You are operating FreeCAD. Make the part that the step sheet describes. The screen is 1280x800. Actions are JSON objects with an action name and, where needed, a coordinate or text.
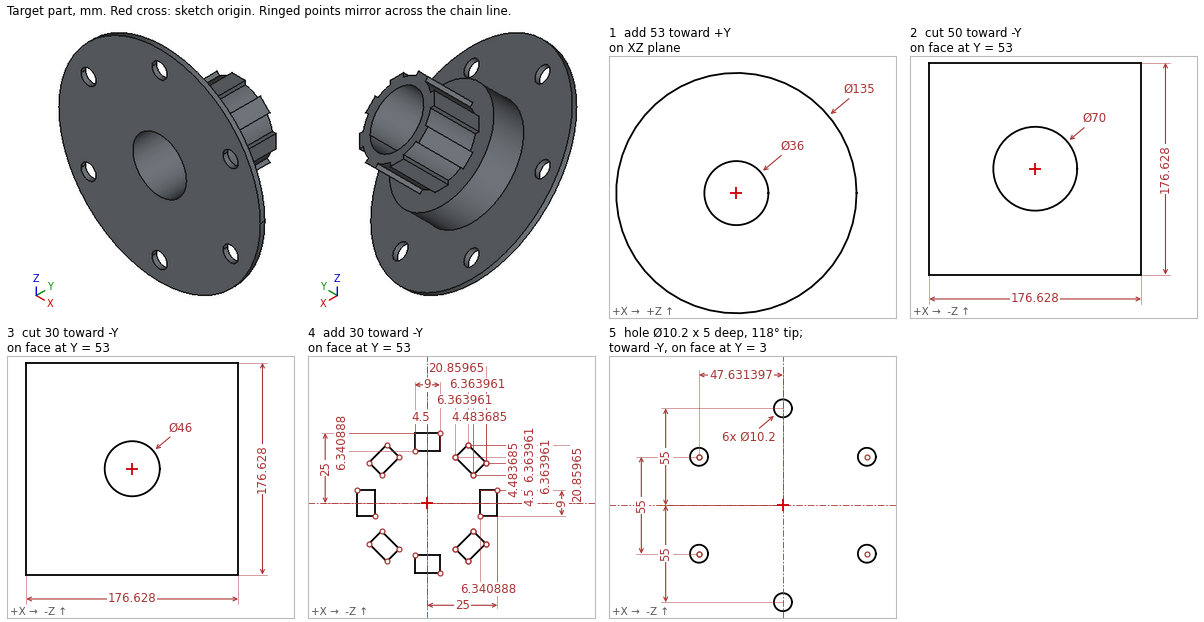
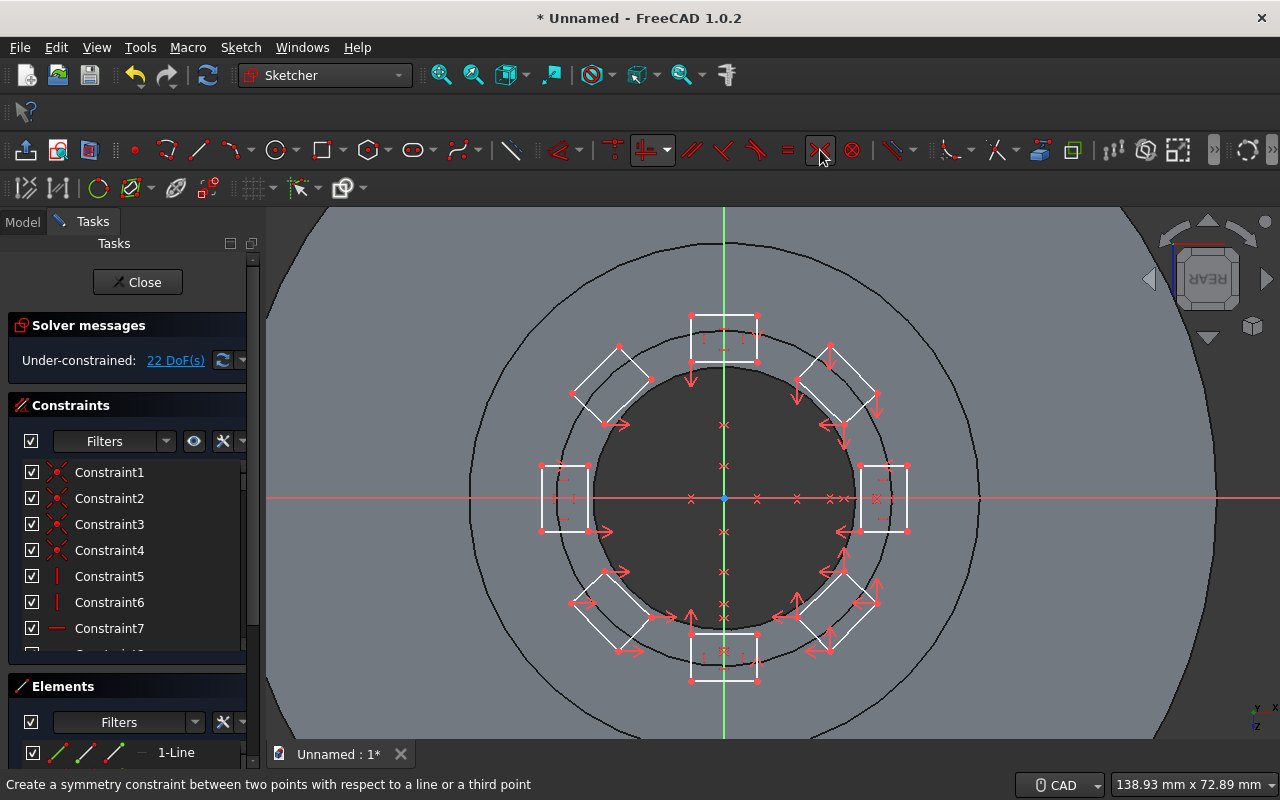
{"action": "left_click", "coordinate": [797, 379]}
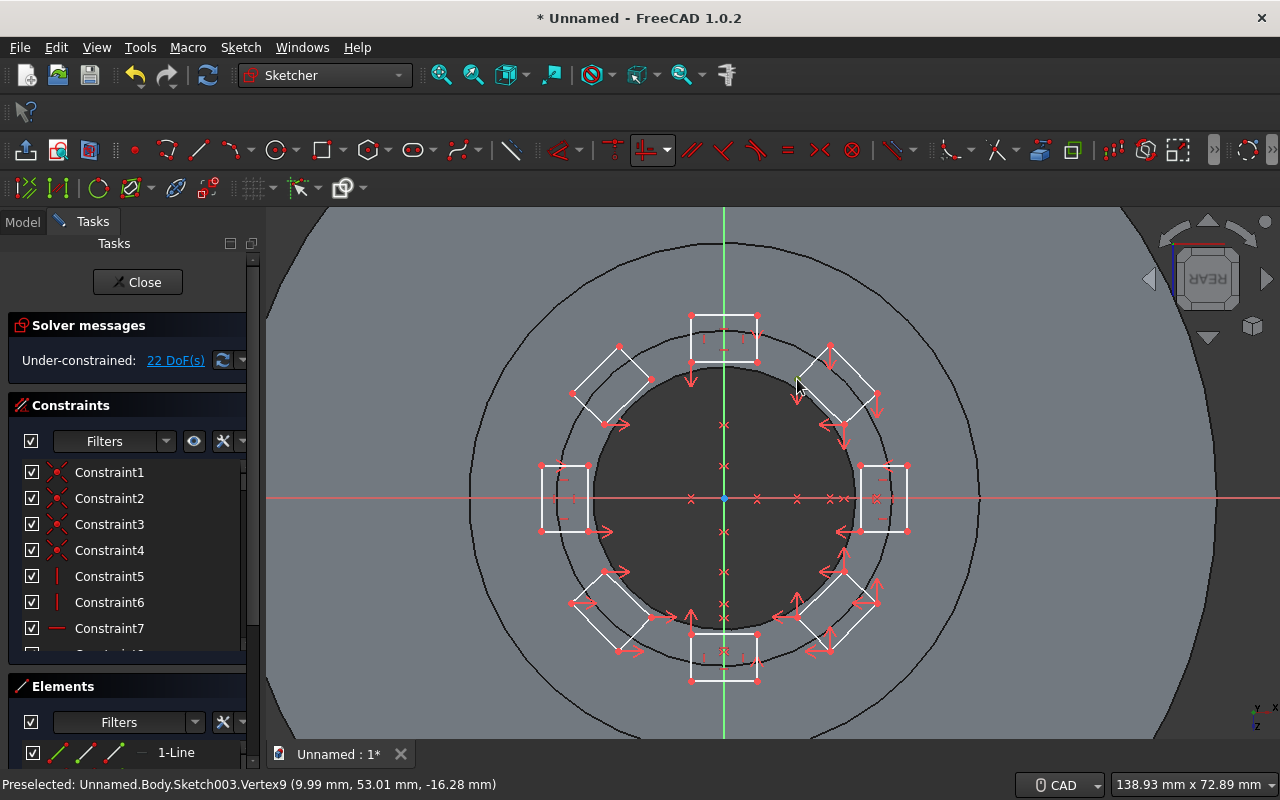
{"action": "left_click", "coordinate": [651, 380]}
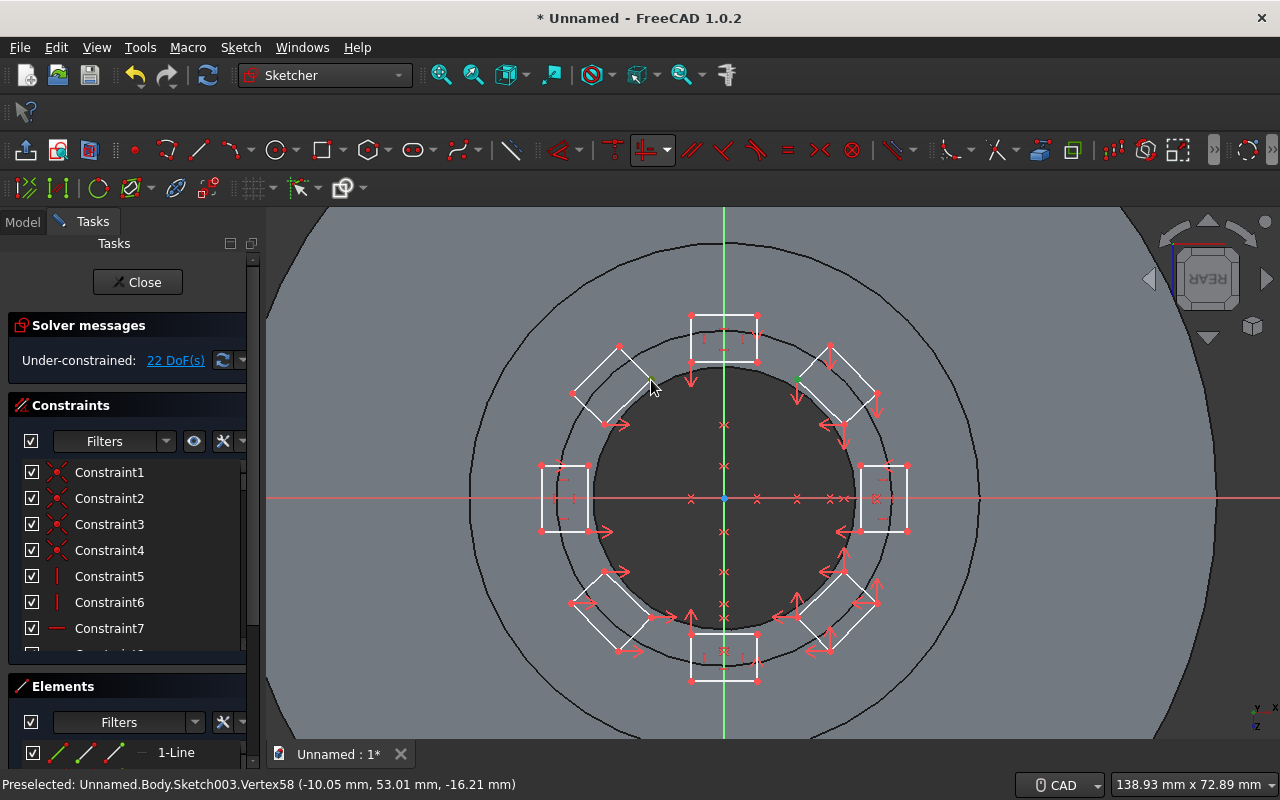
{"action": "left_click", "coordinate": [724, 541]}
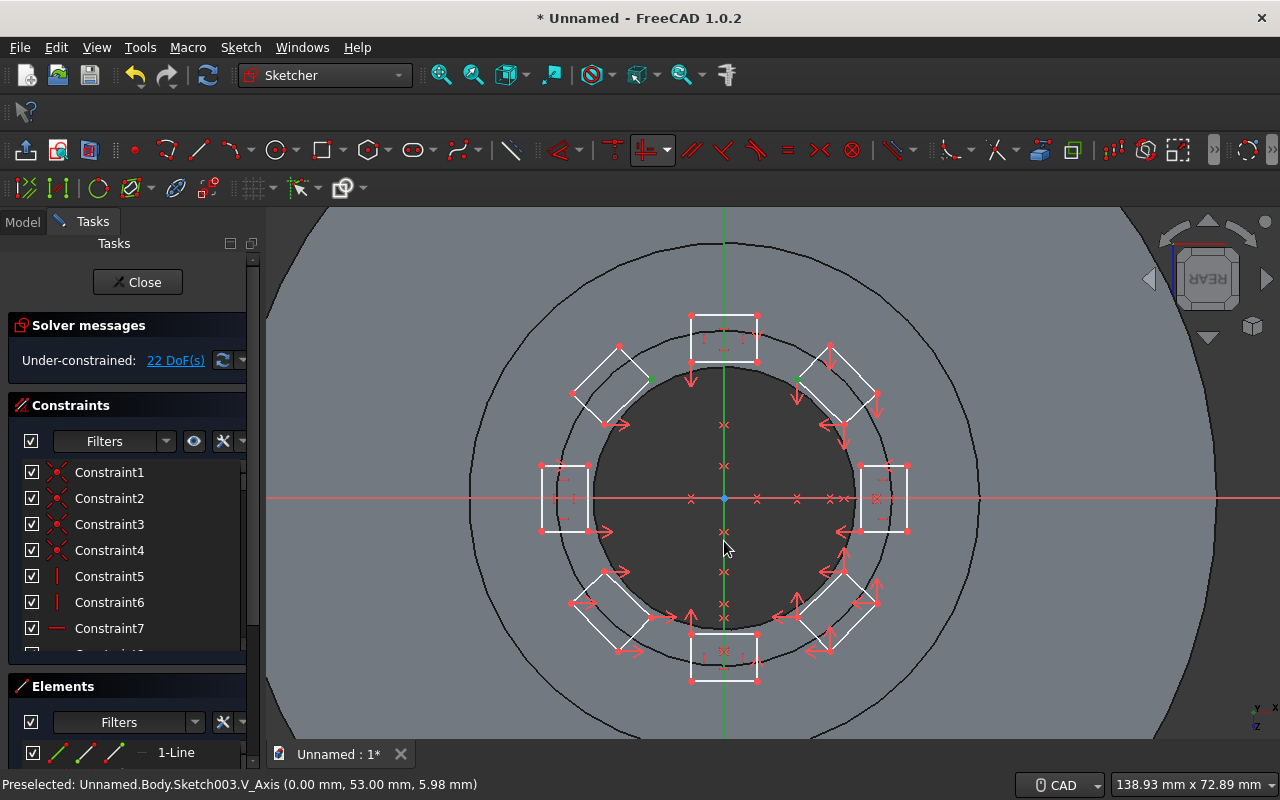
{"action": "left_click", "coordinate": [820, 150]}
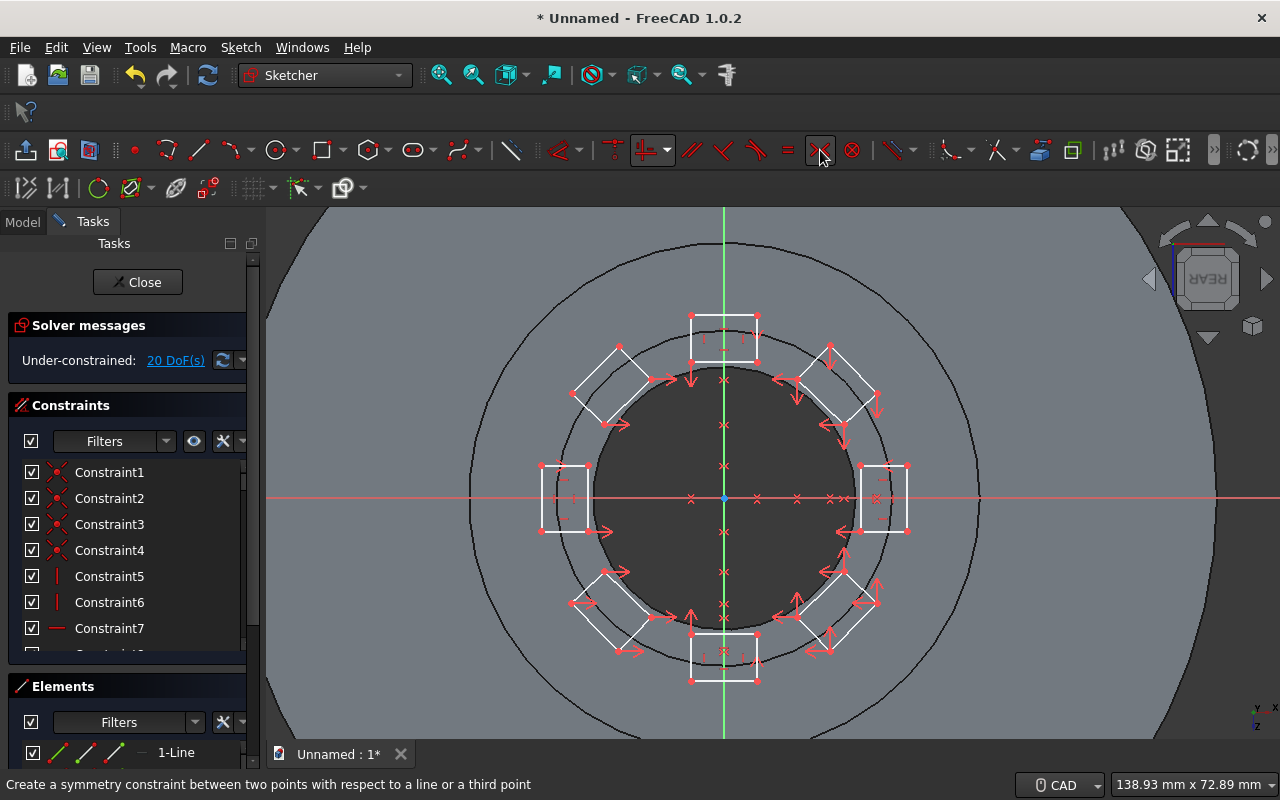
{"action": "left_click", "coordinate": [830, 345]}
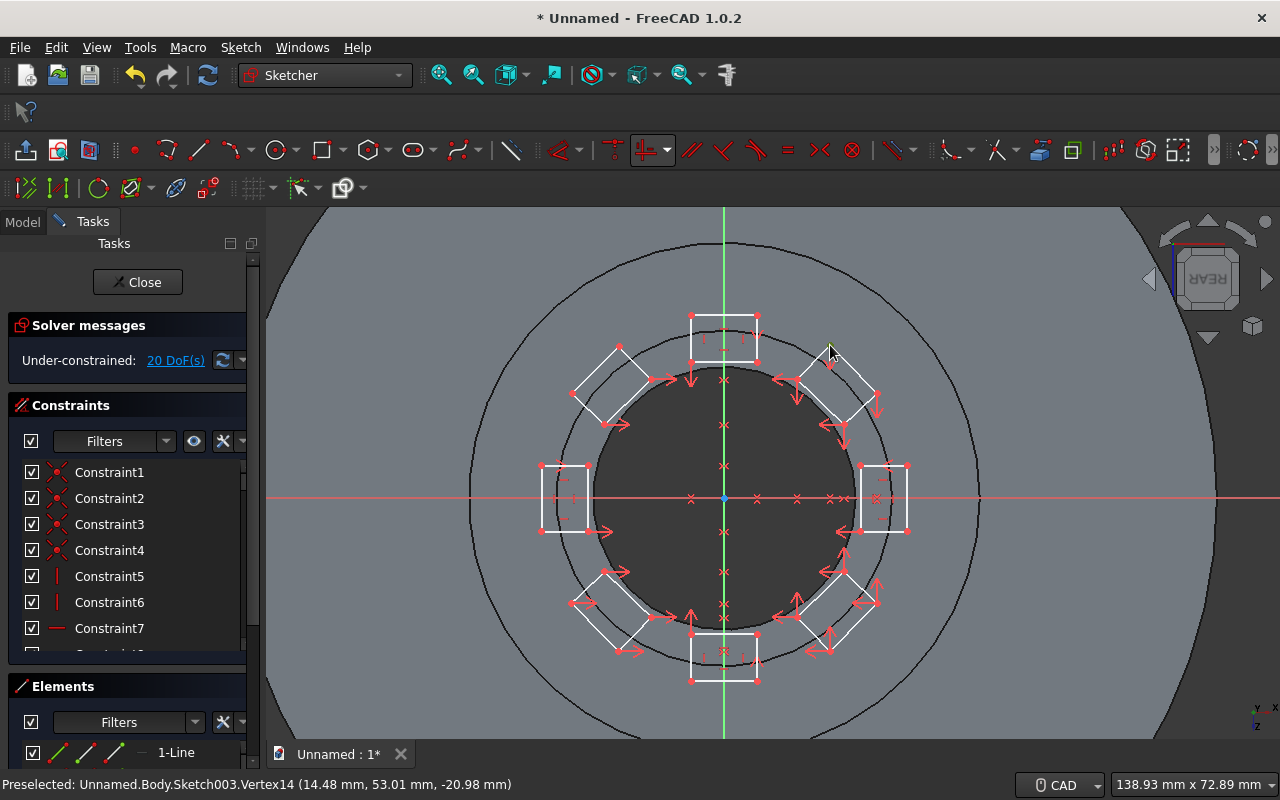
{"action": "left_click", "coordinate": [619, 347]}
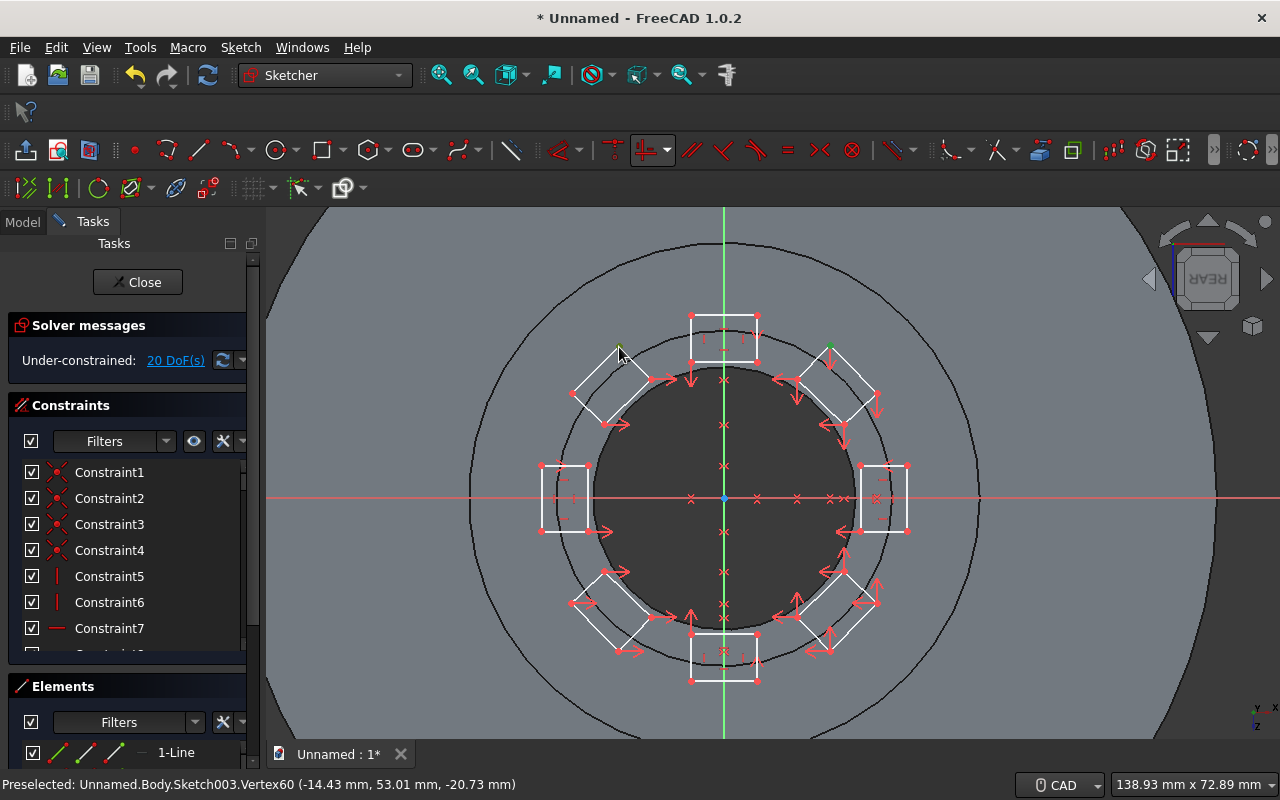
{"action": "left_click", "coordinate": [724, 541]}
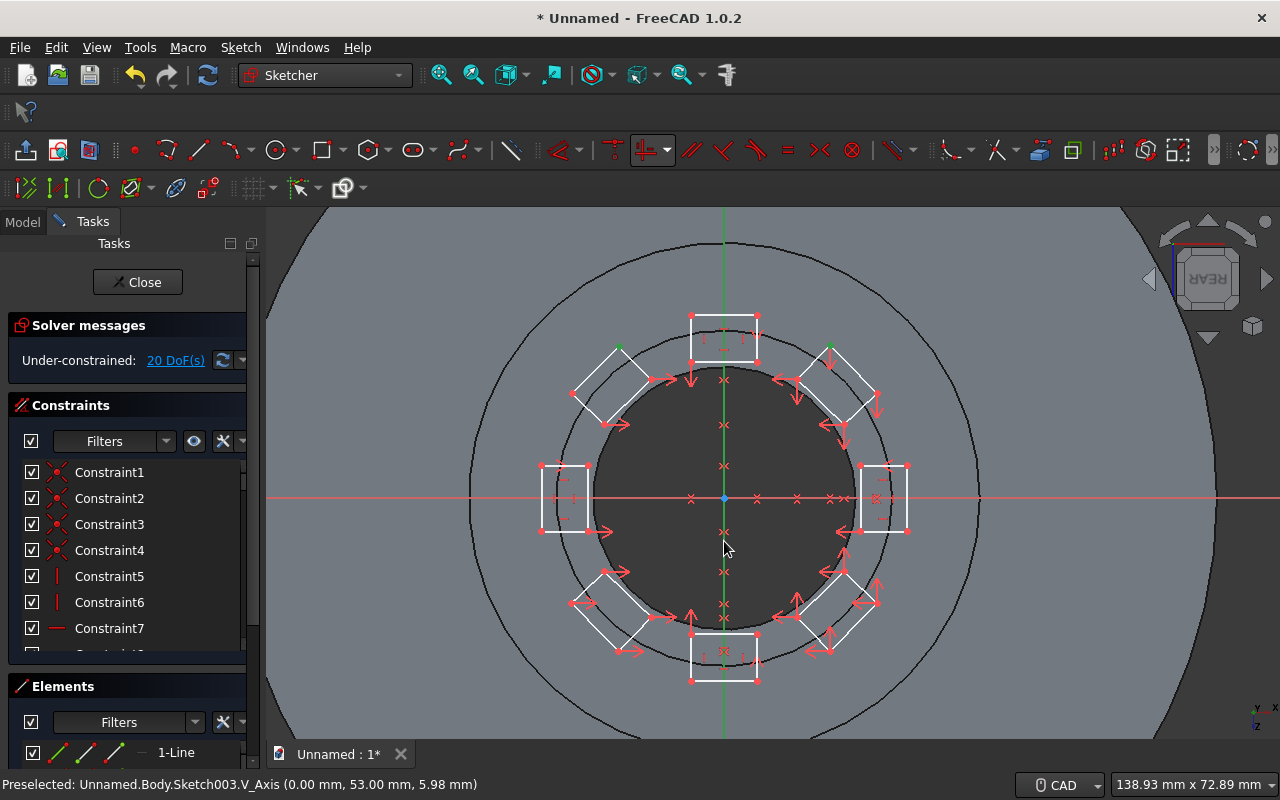
{"action": "left_click", "coordinate": [820, 150]}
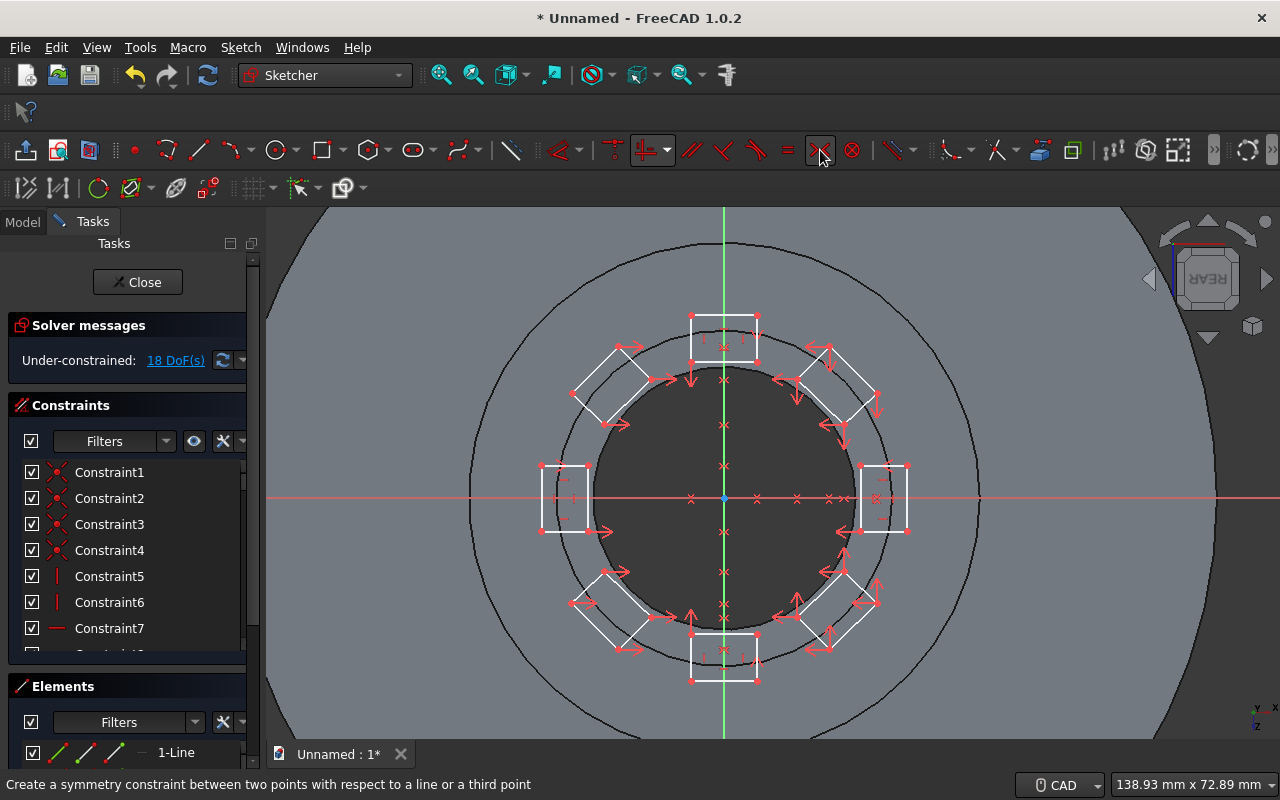
{"action": "left_click", "coordinate": [877, 393]}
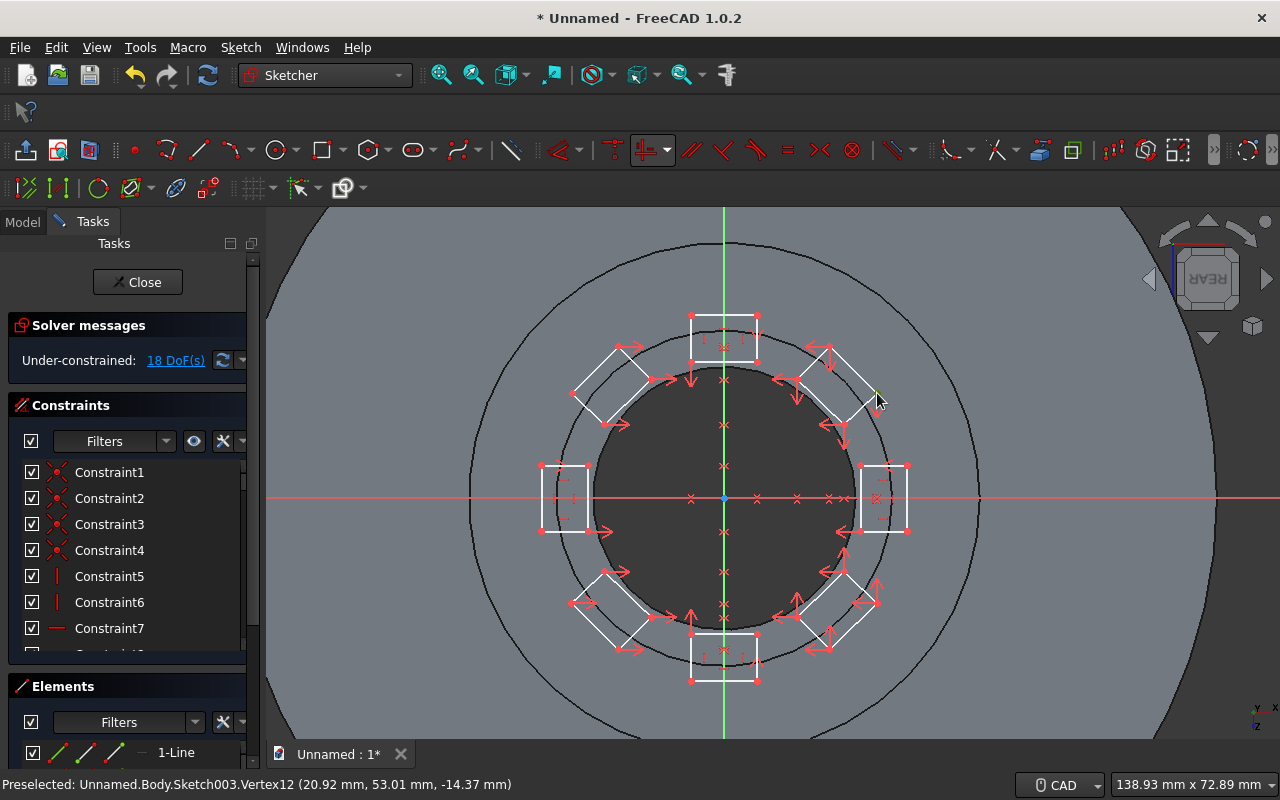
{"action": "left_click", "coordinate": [572, 394]}